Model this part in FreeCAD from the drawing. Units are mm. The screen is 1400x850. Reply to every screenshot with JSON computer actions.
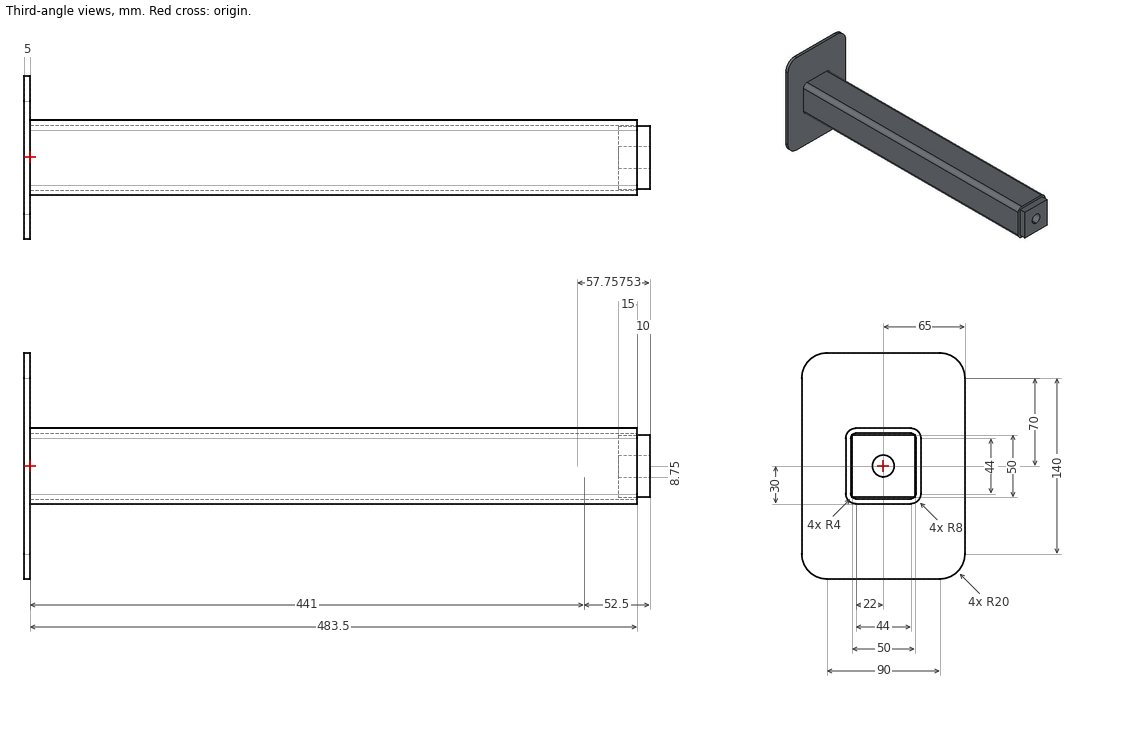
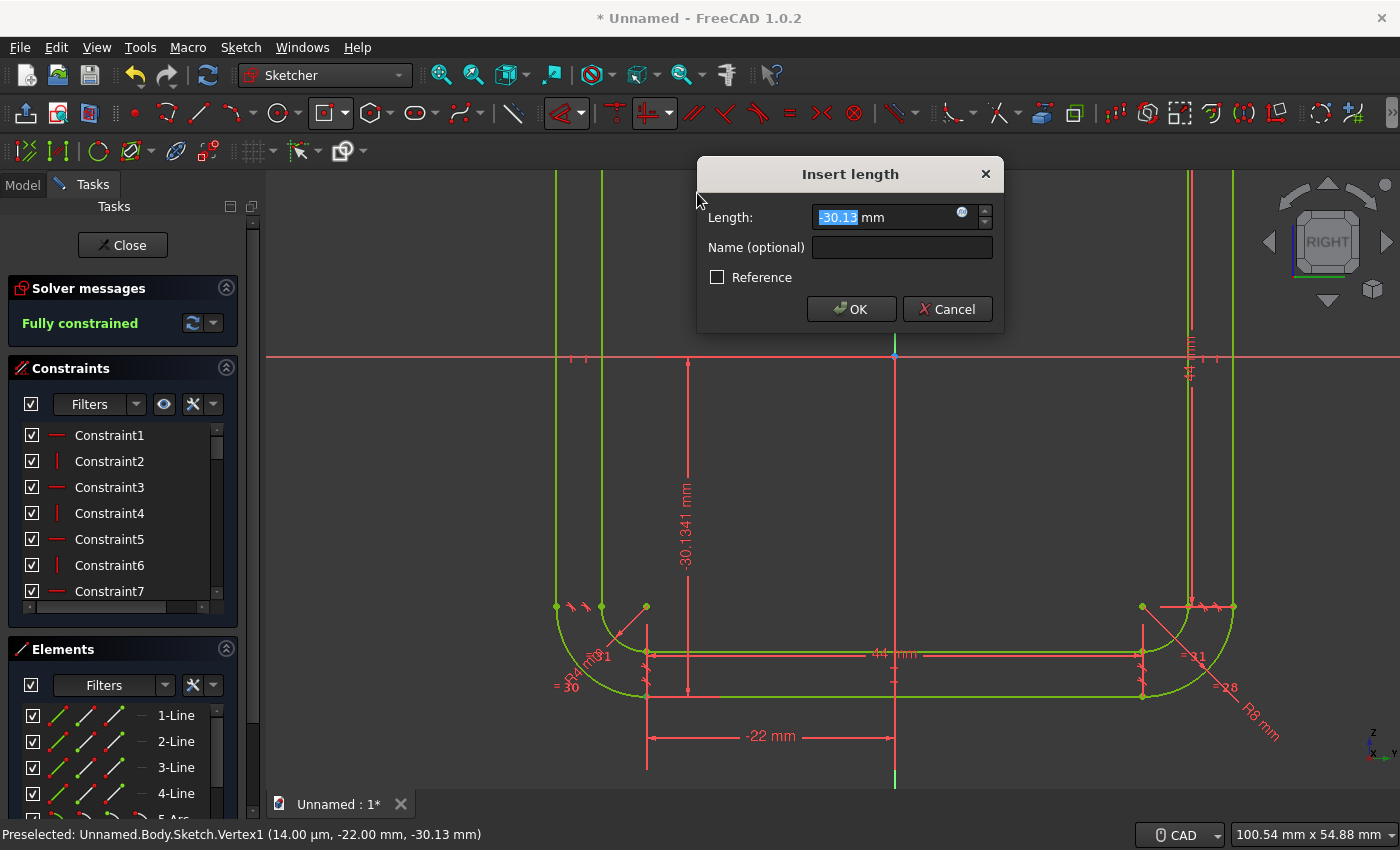
{"action": "type", "text": "-30"}
{"action": "key", "text": "Return"}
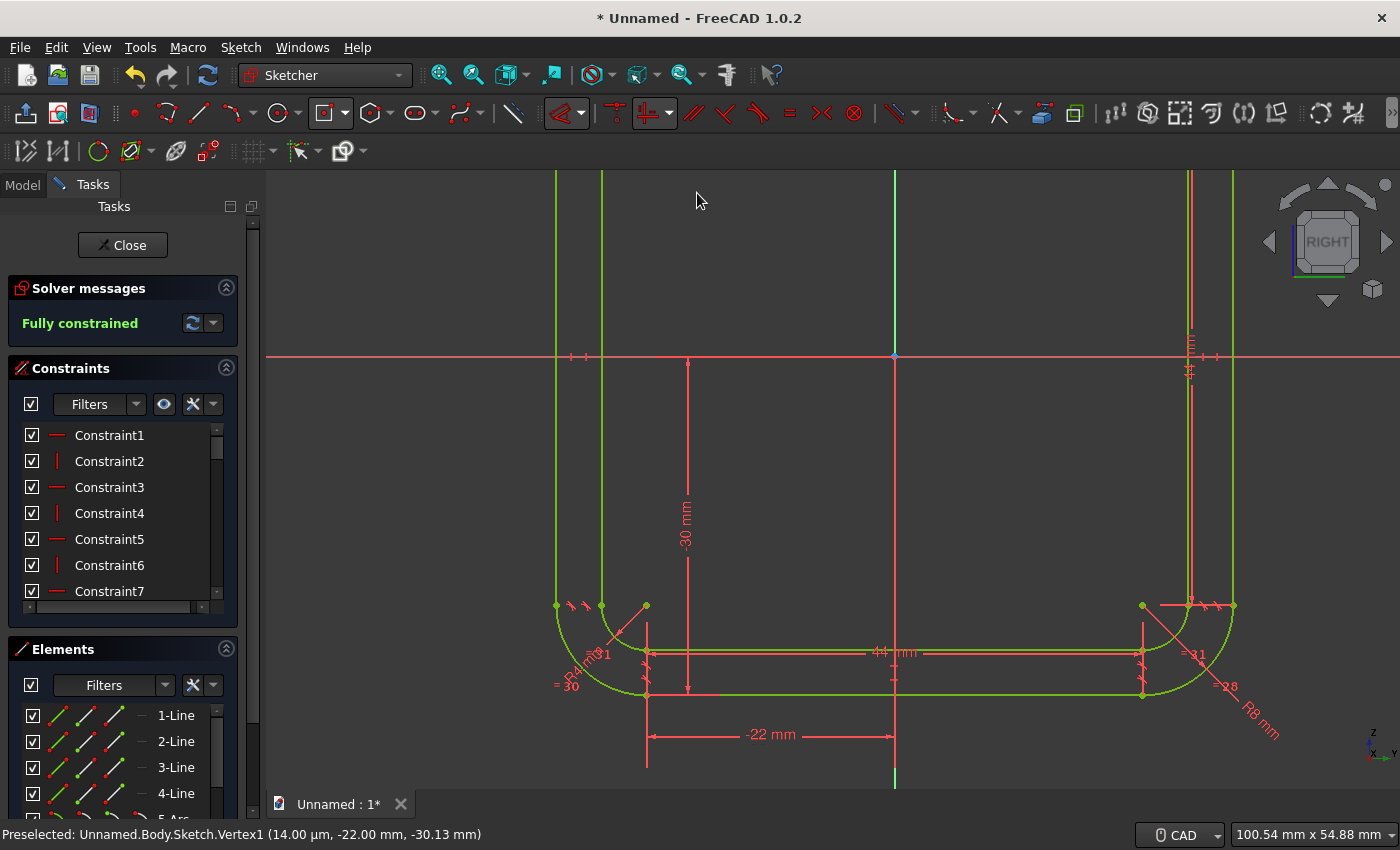
{"action": "left_click", "coordinate": [123, 245]}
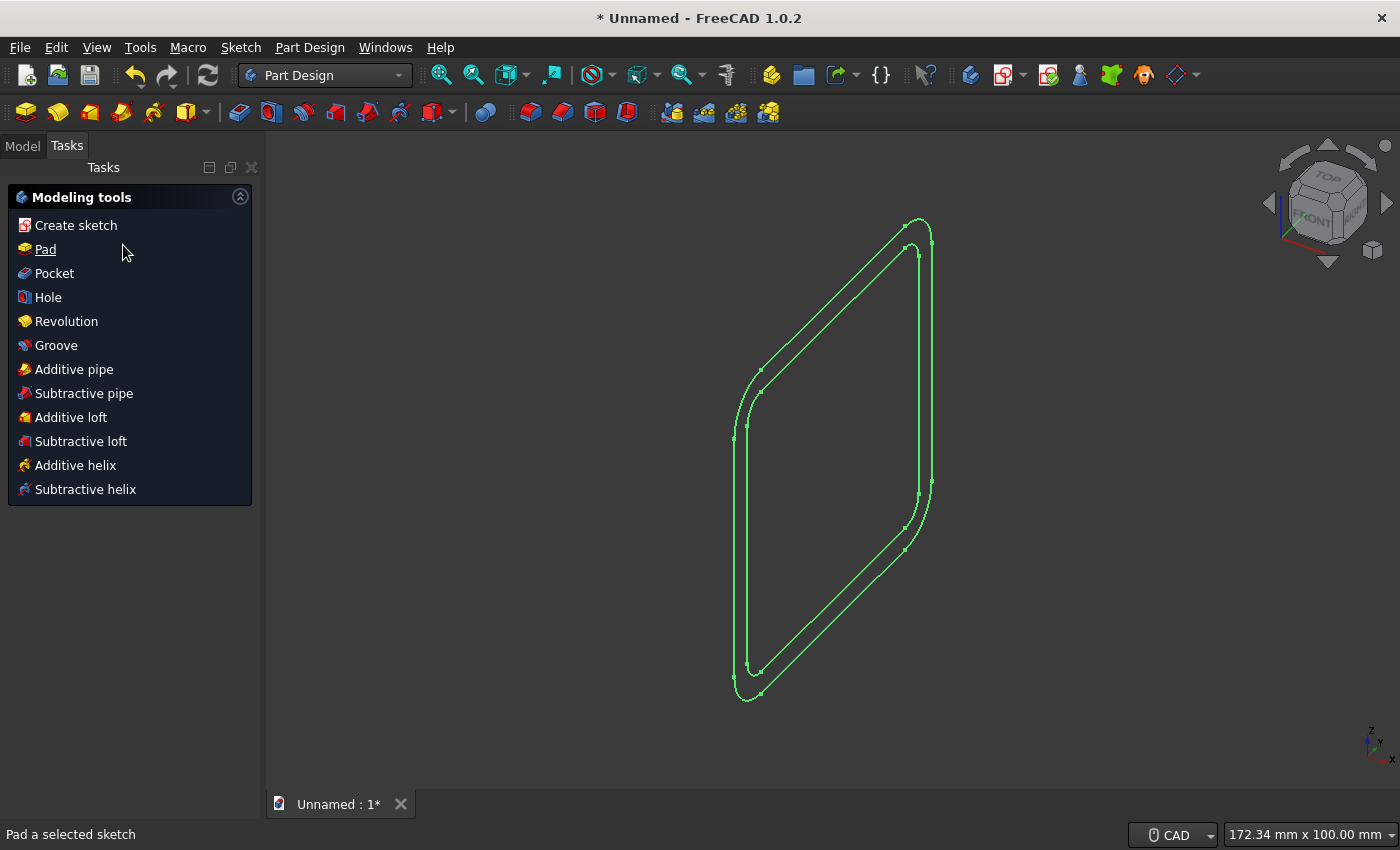
{"action": "left_click", "coordinate": [26, 112]}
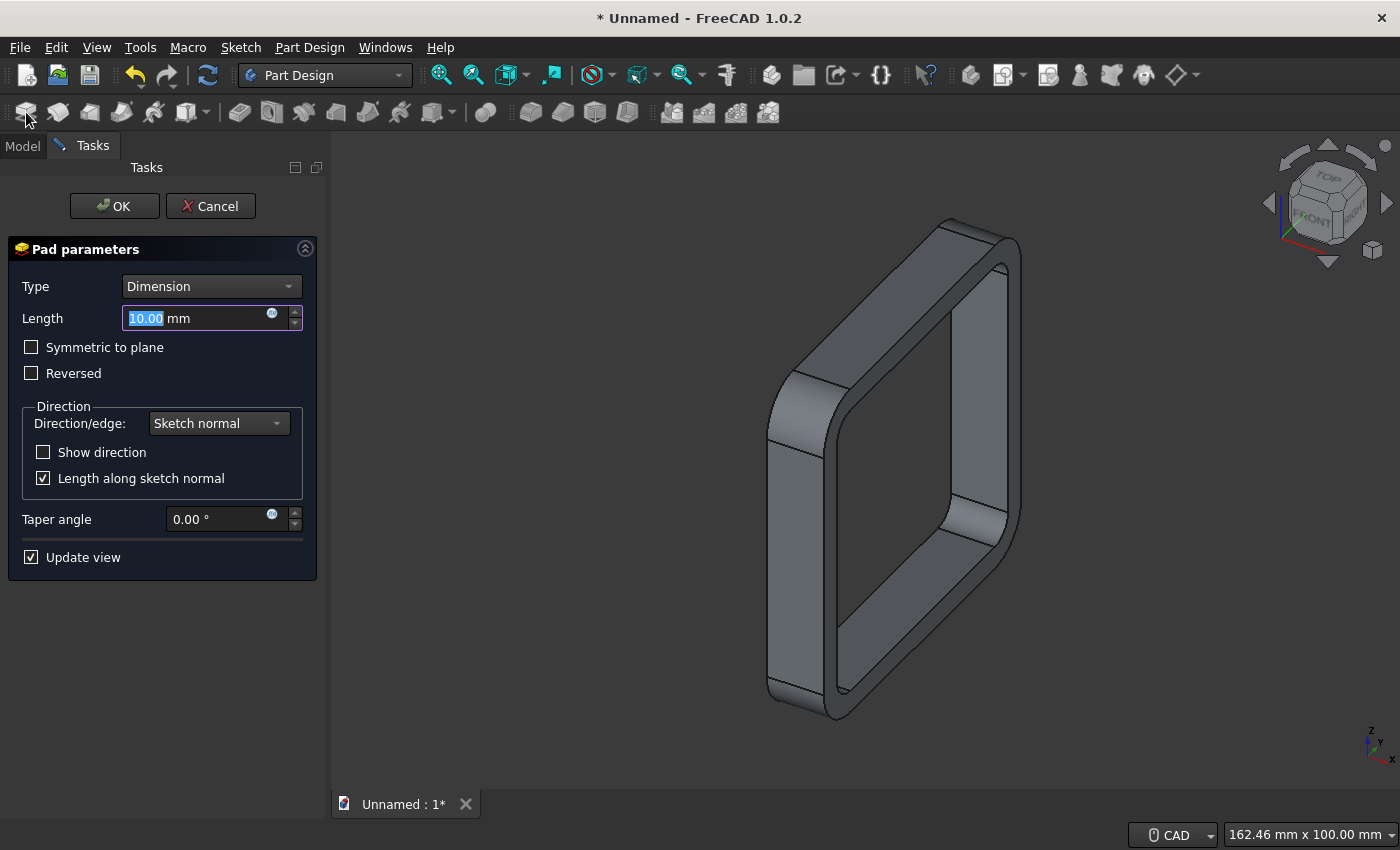
{"action": "type", "text": "483.5"}
{"action": "key", "text": "Tab"}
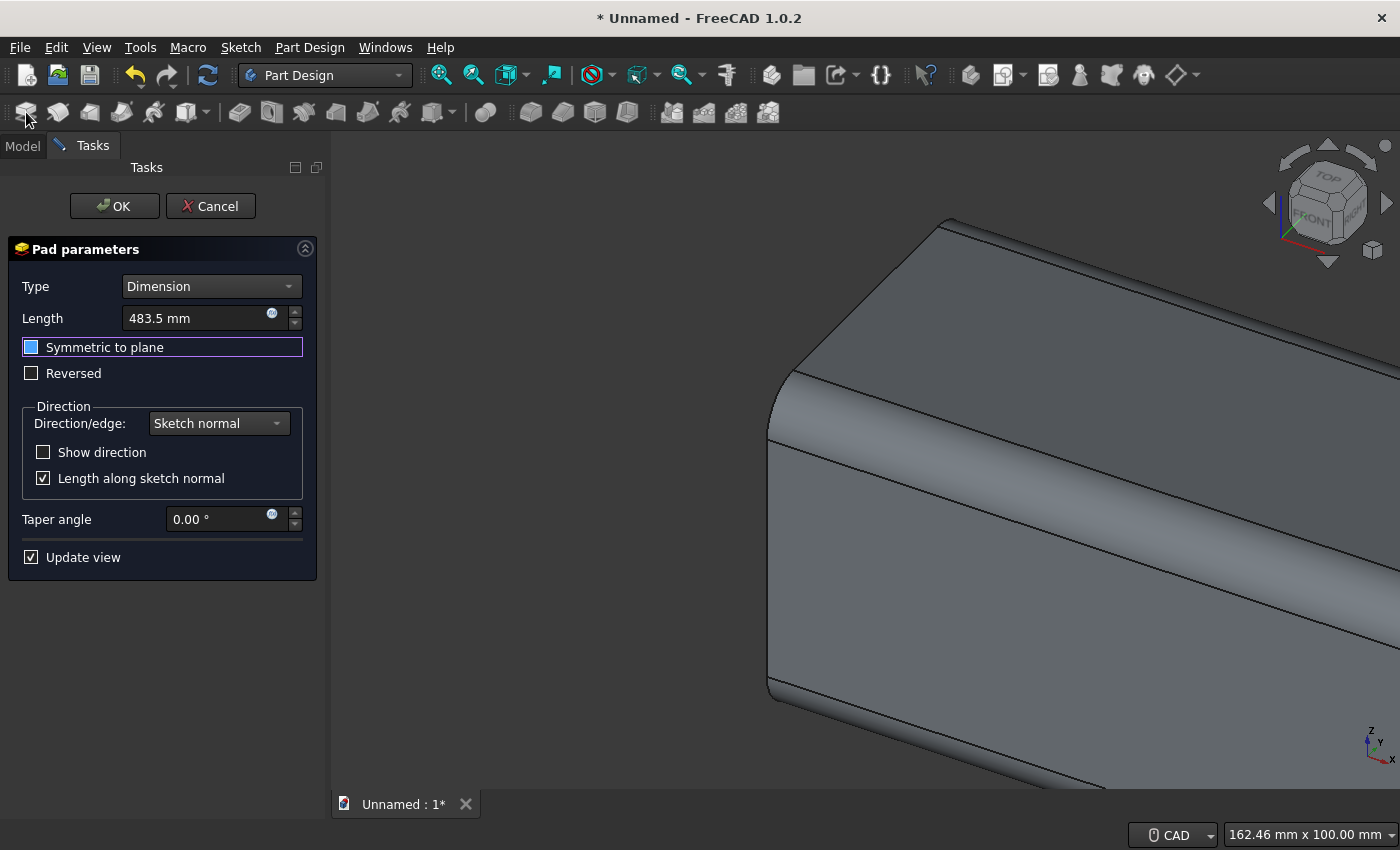
{"action": "left_click", "coordinate": [115, 206]}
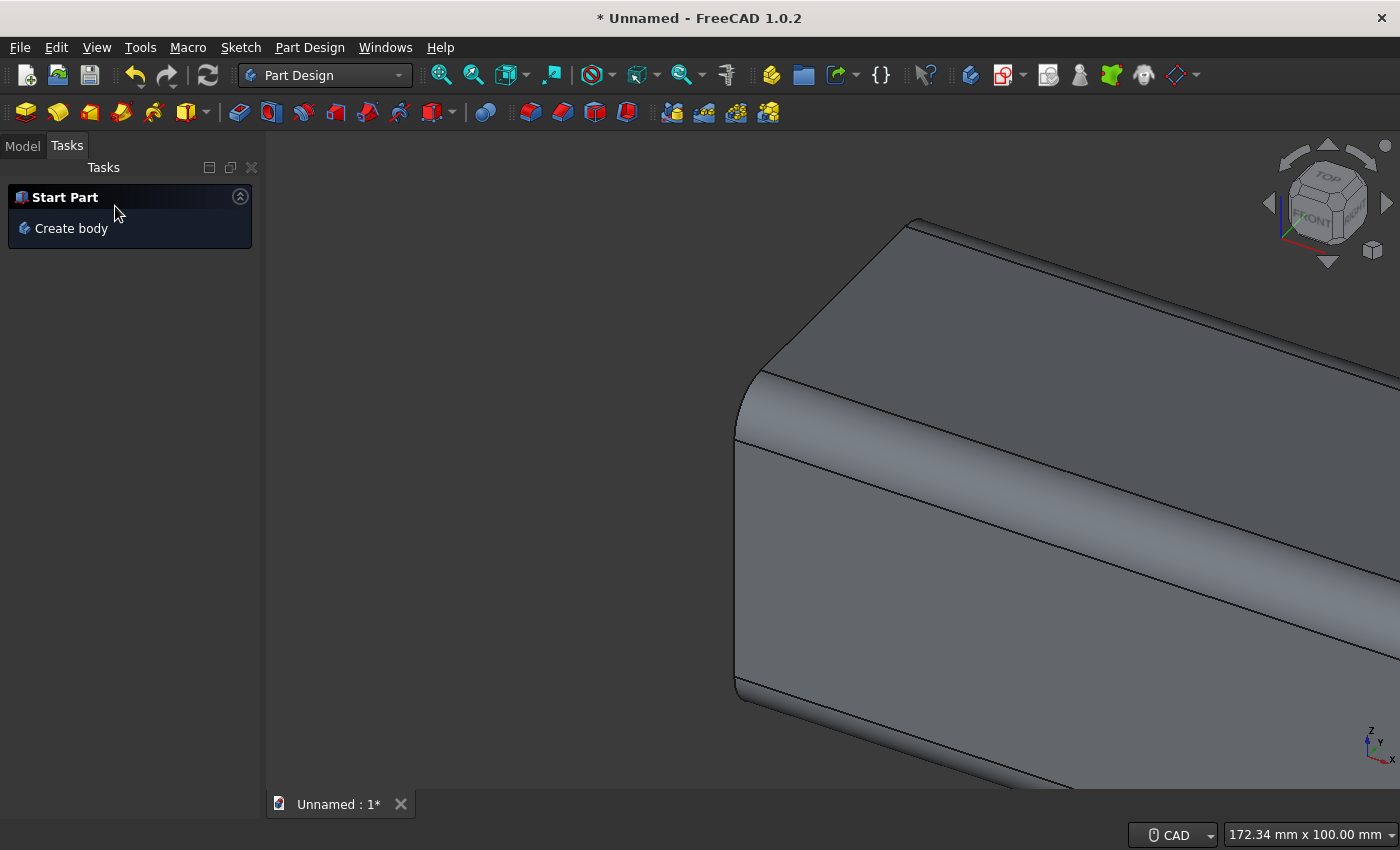
{"action": "left_click", "coordinate": [442, 76]}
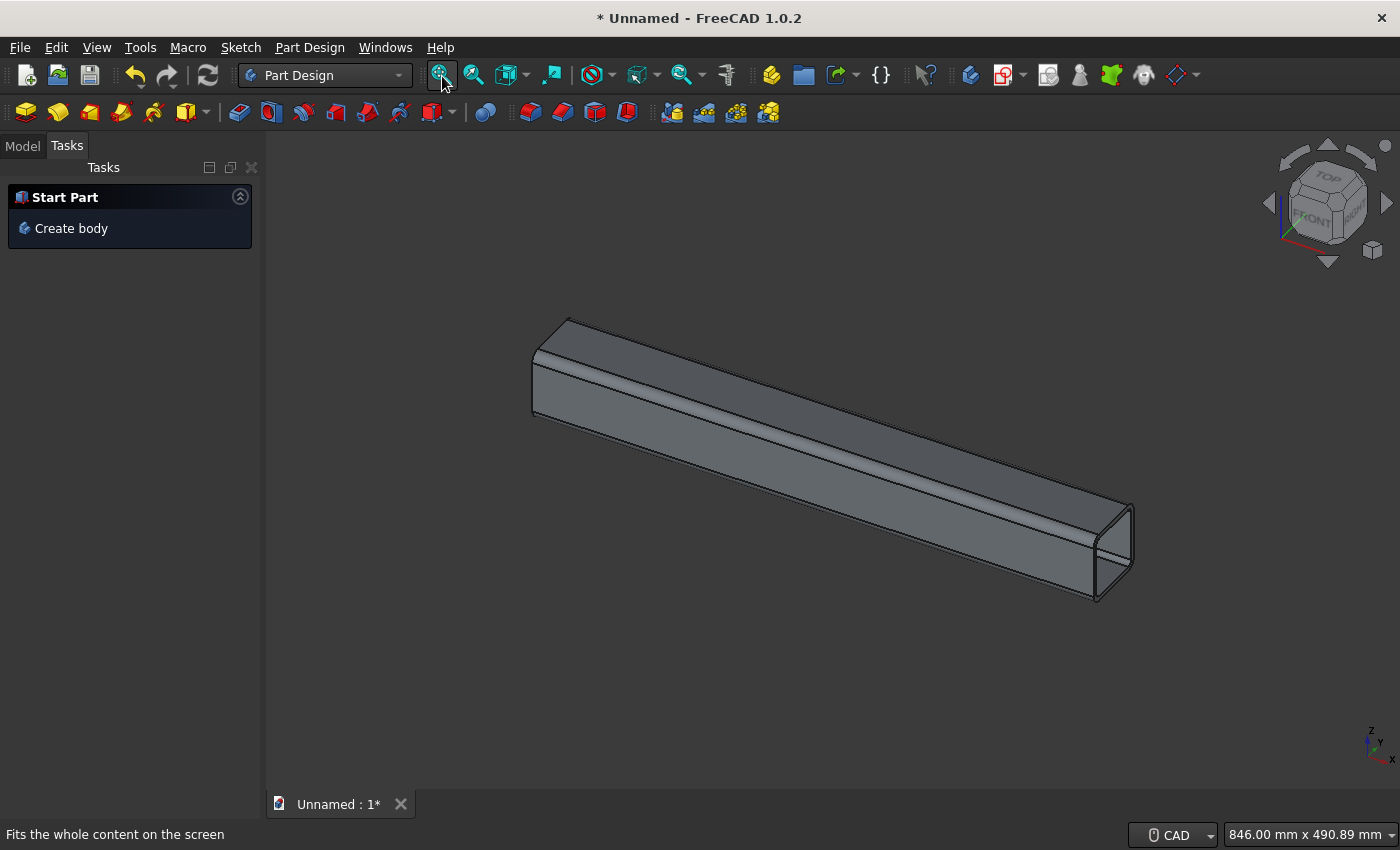
{"action": "left_click", "coordinate": [972, 76]}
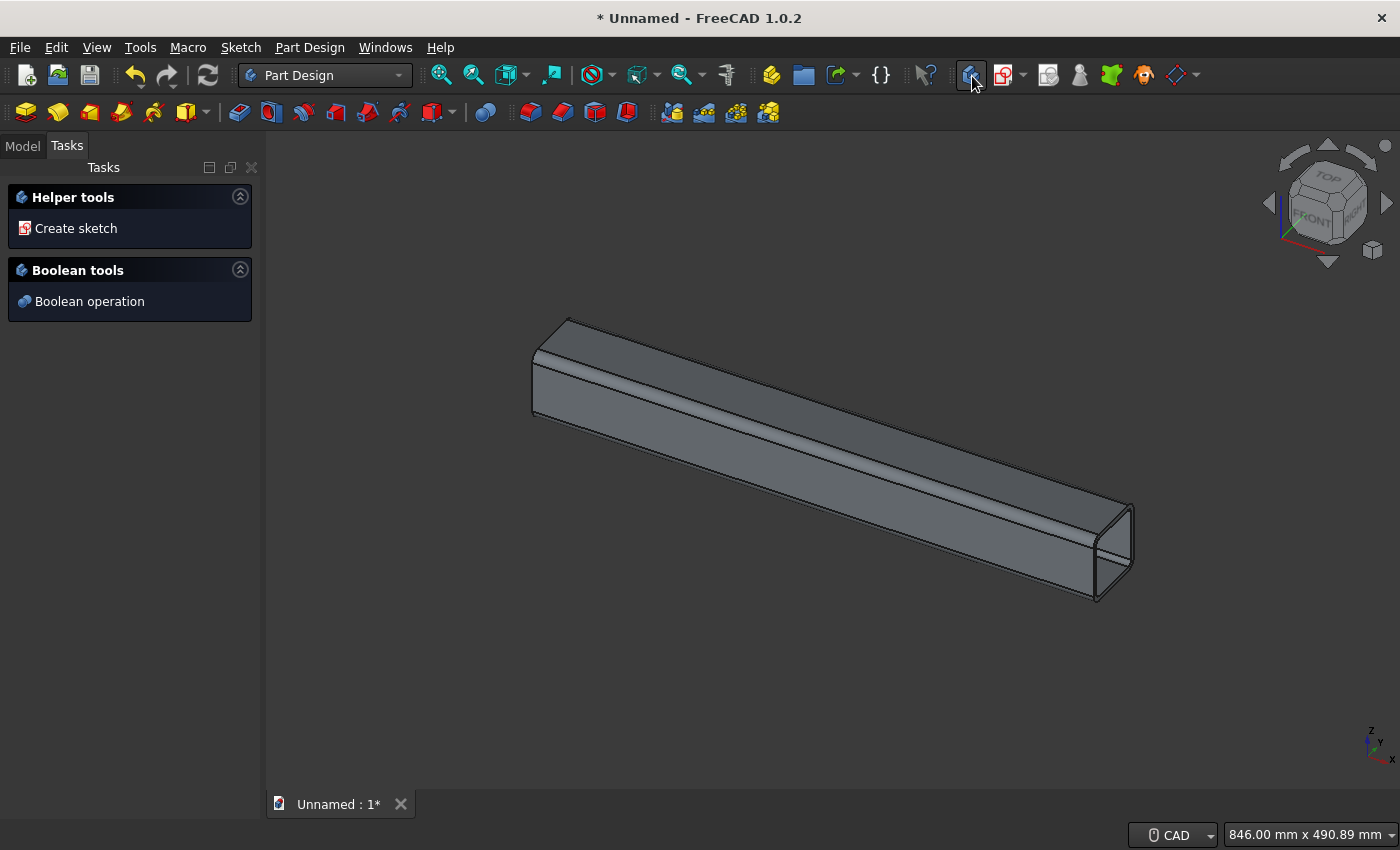
{"action": "left_click", "coordinate": [306, 749]}